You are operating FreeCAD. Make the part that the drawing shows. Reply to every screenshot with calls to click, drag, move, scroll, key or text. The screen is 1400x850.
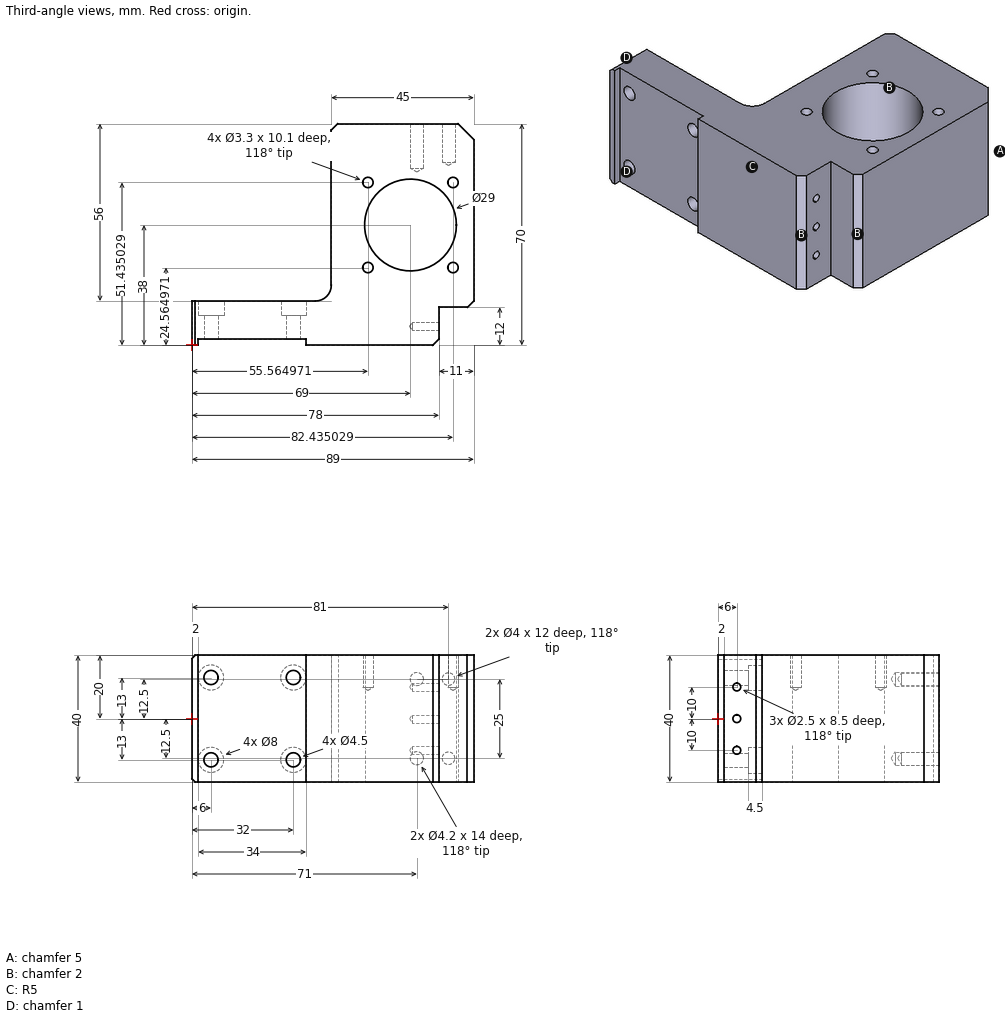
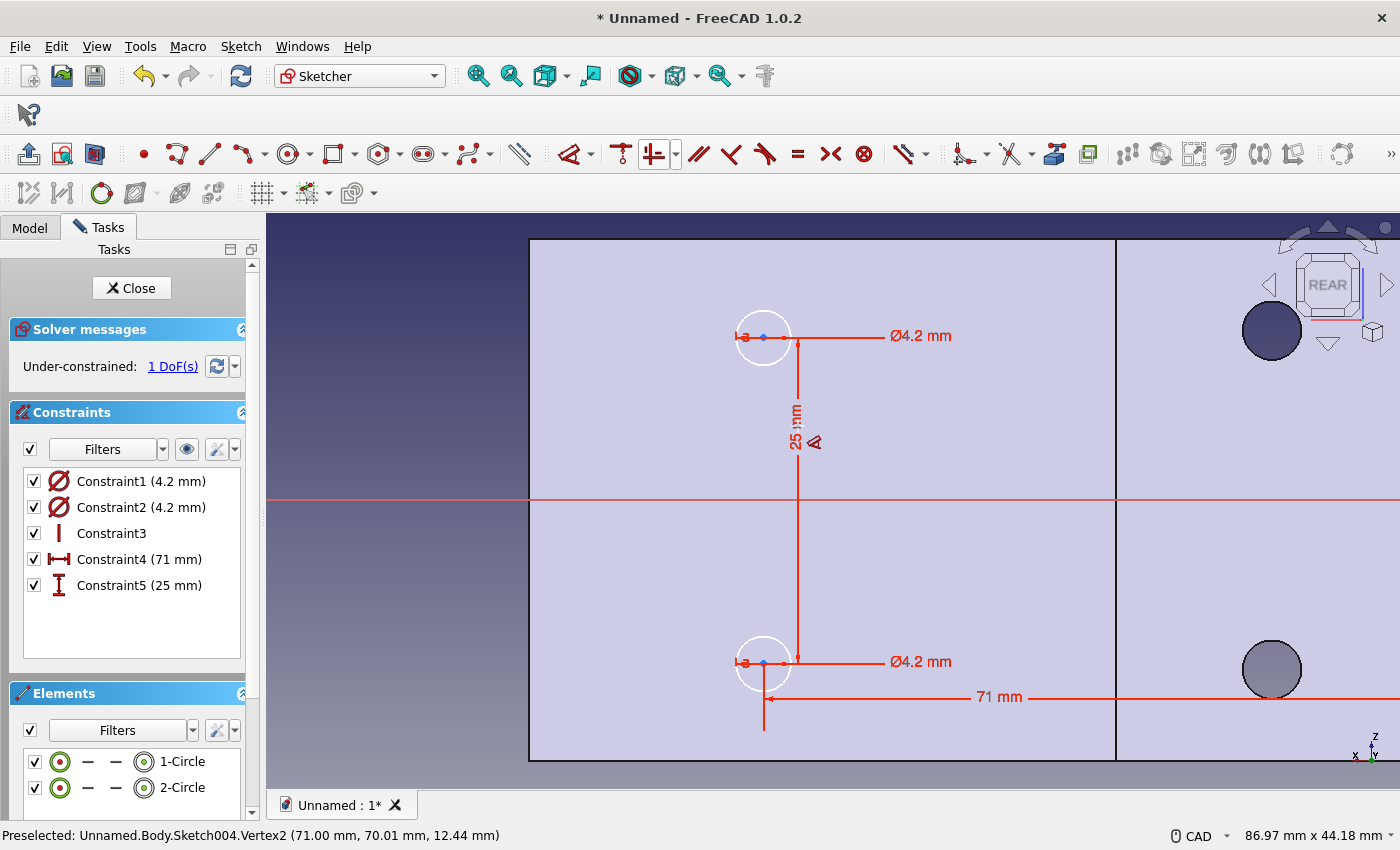
click(764, 664)
click(730, 582)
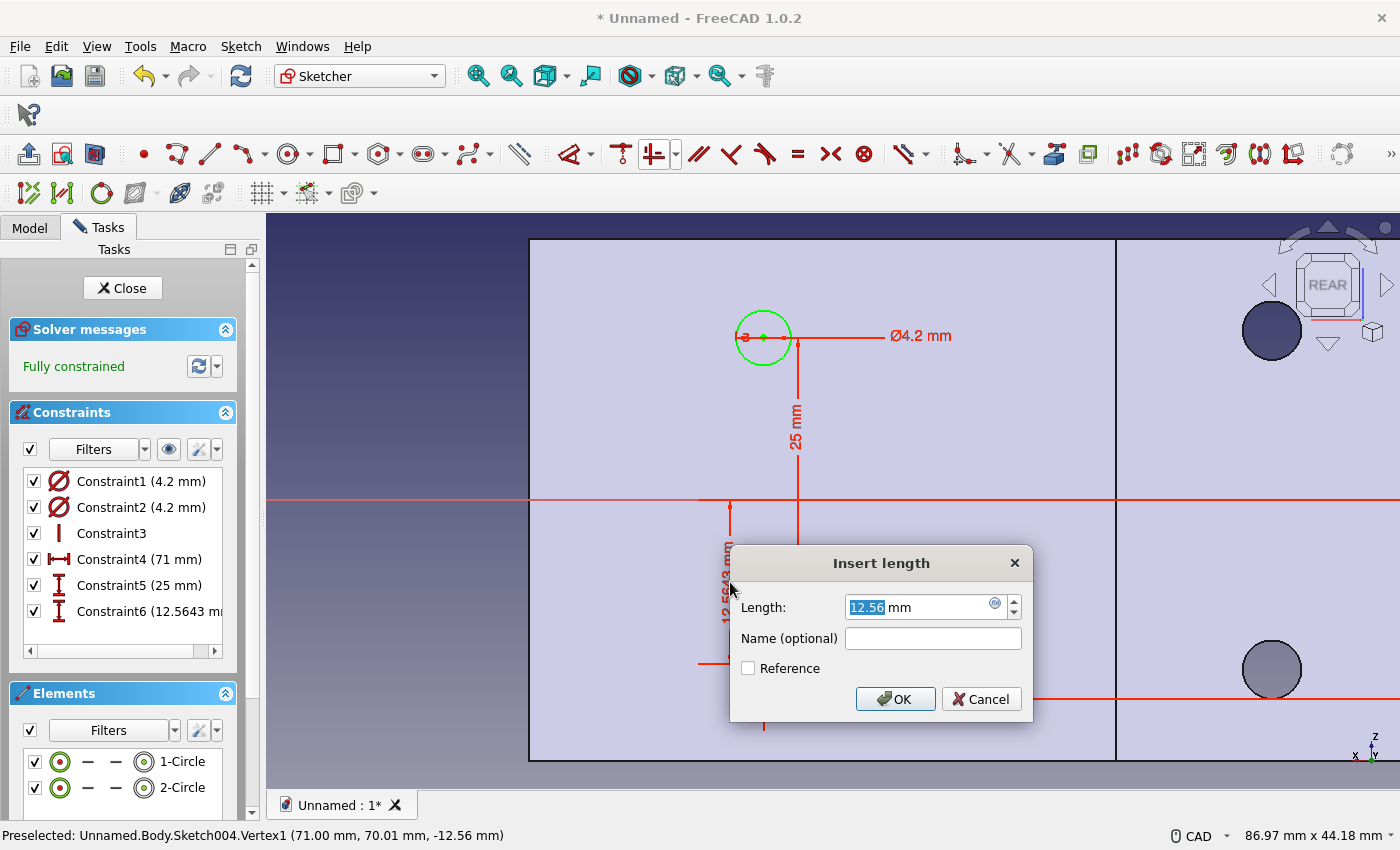
text(12.5)
key(Return)
key(Escape)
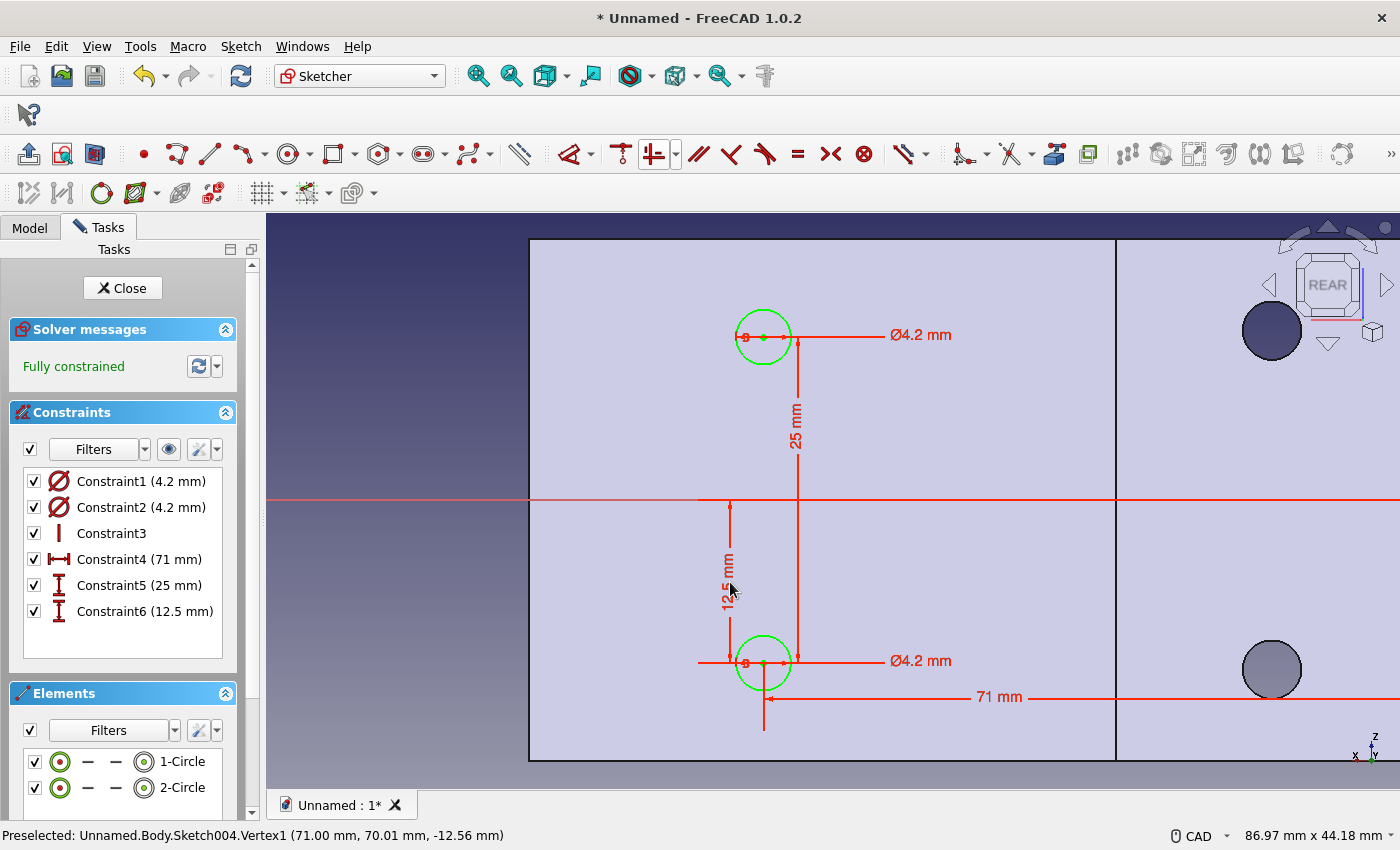
click(123, 288)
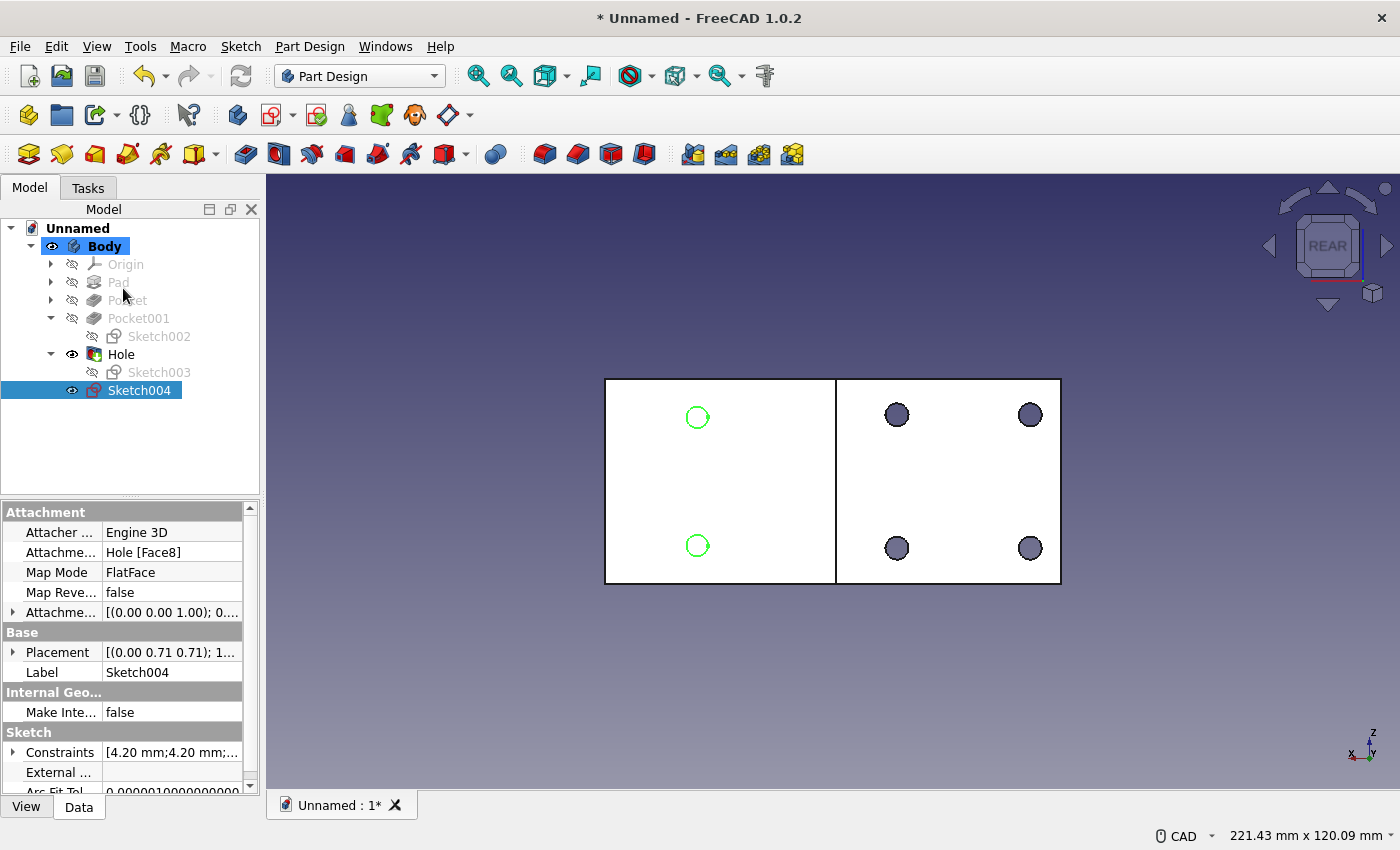
click(279, 154)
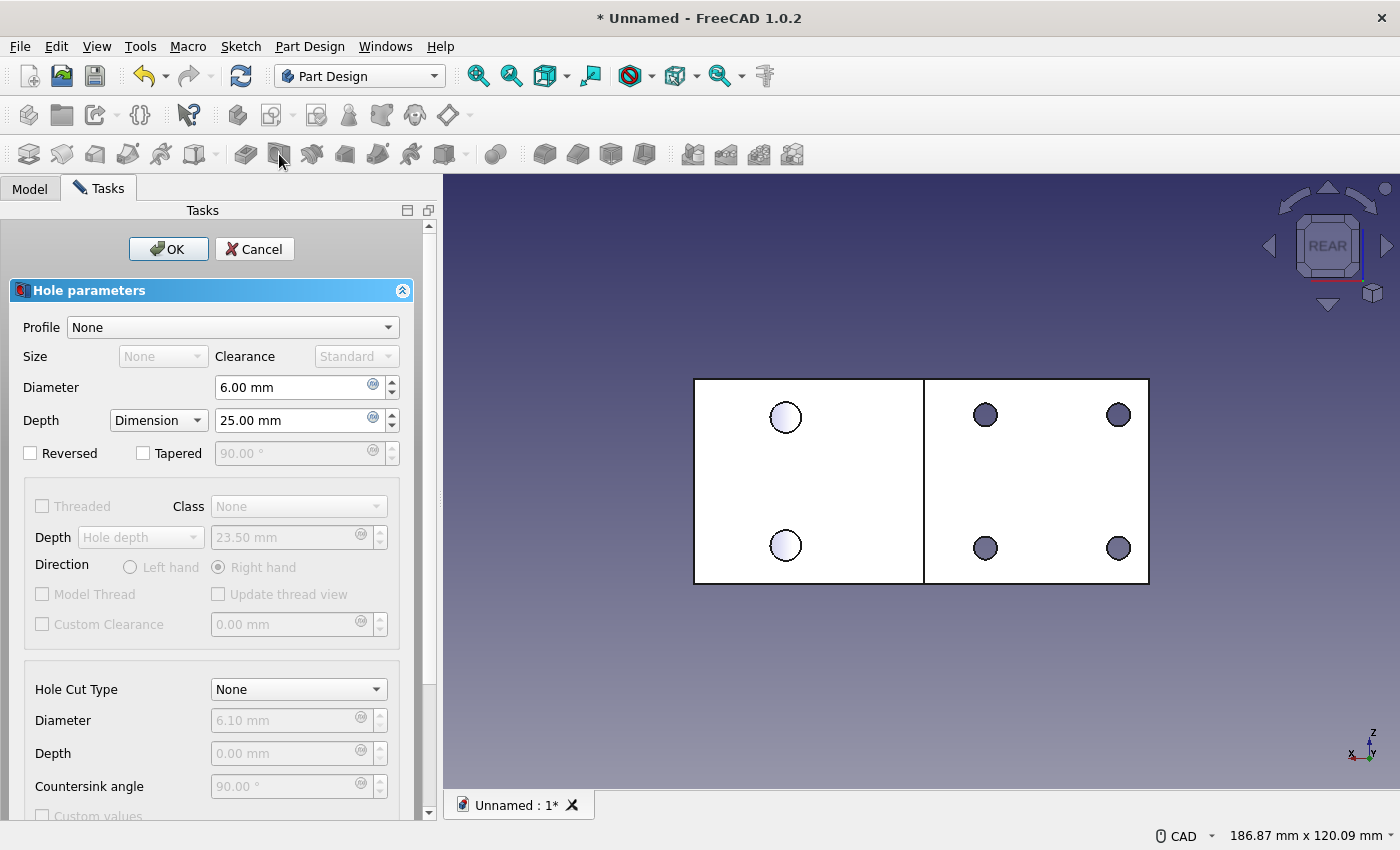
triple_click(300, 388)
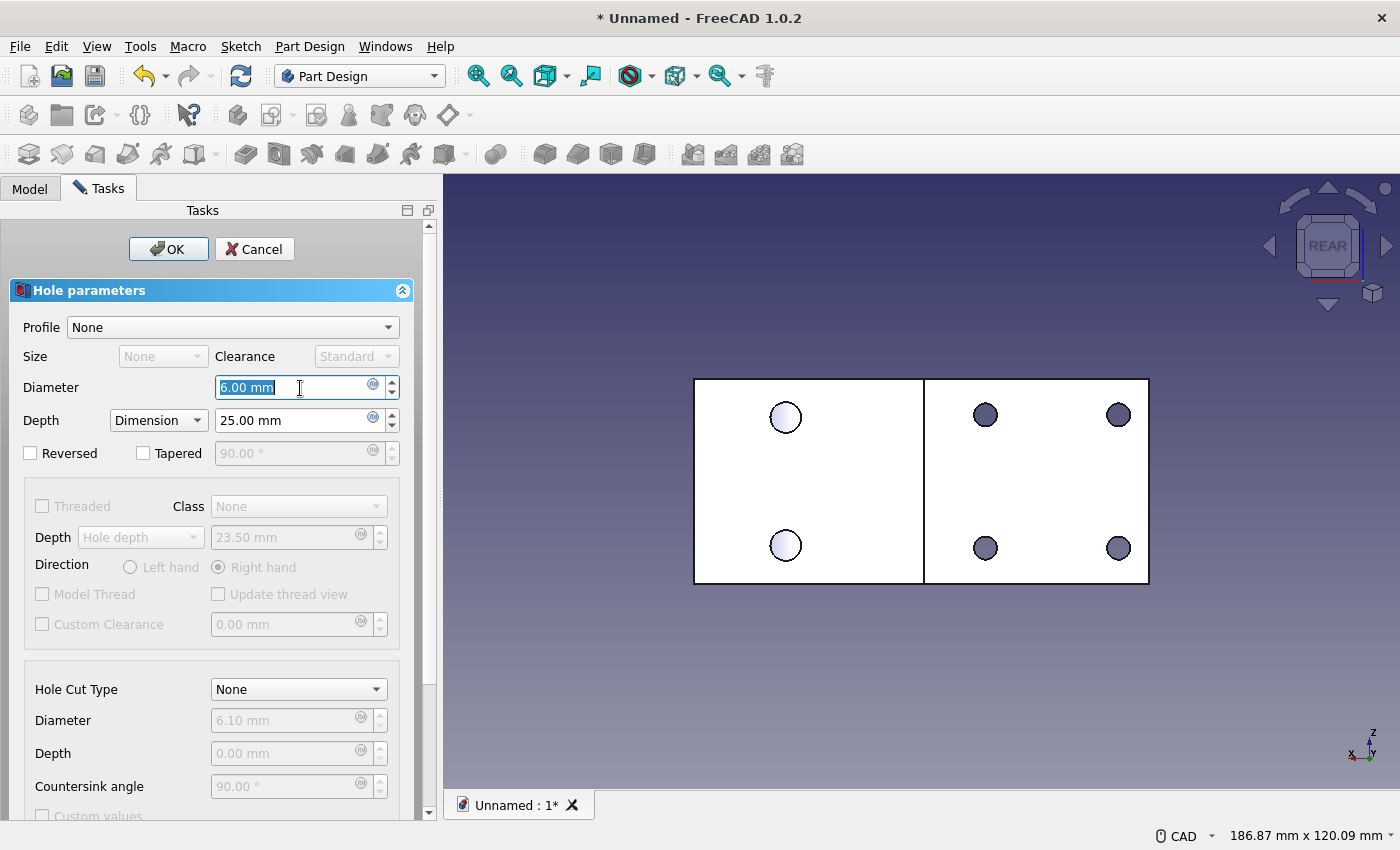
text(4.2)
key(Tab)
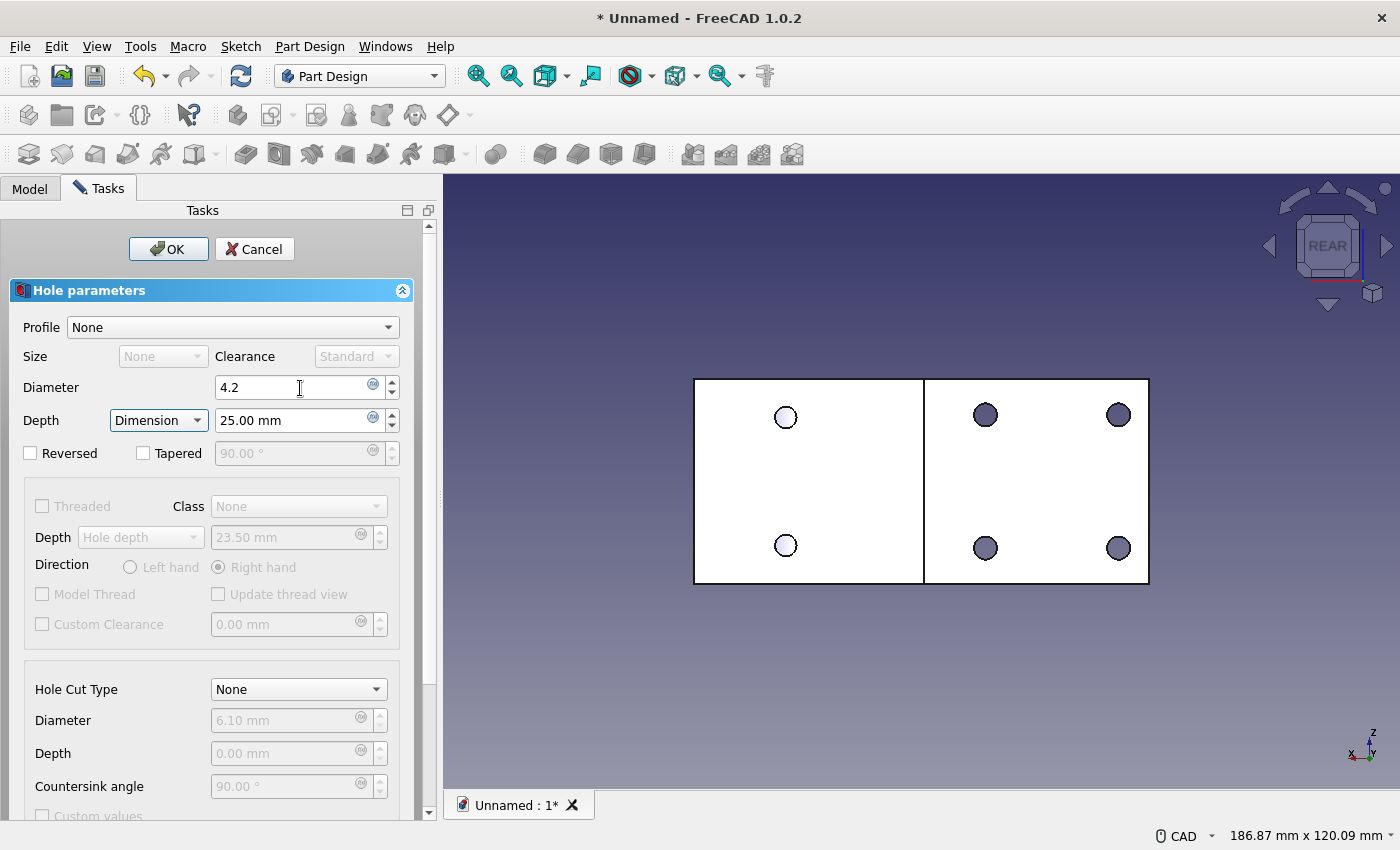
triple_click(300, 420)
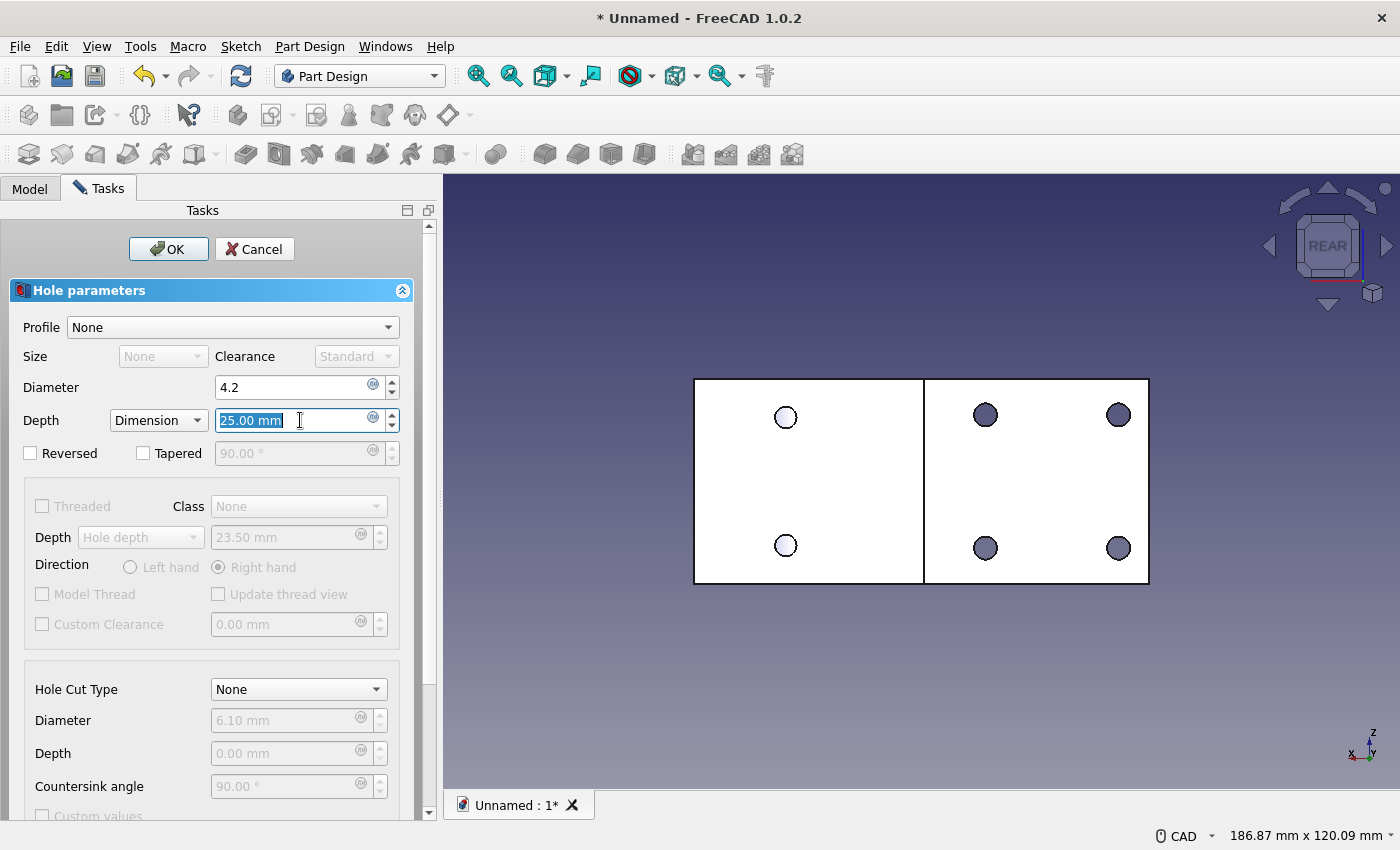
text(14)
key(Tab)